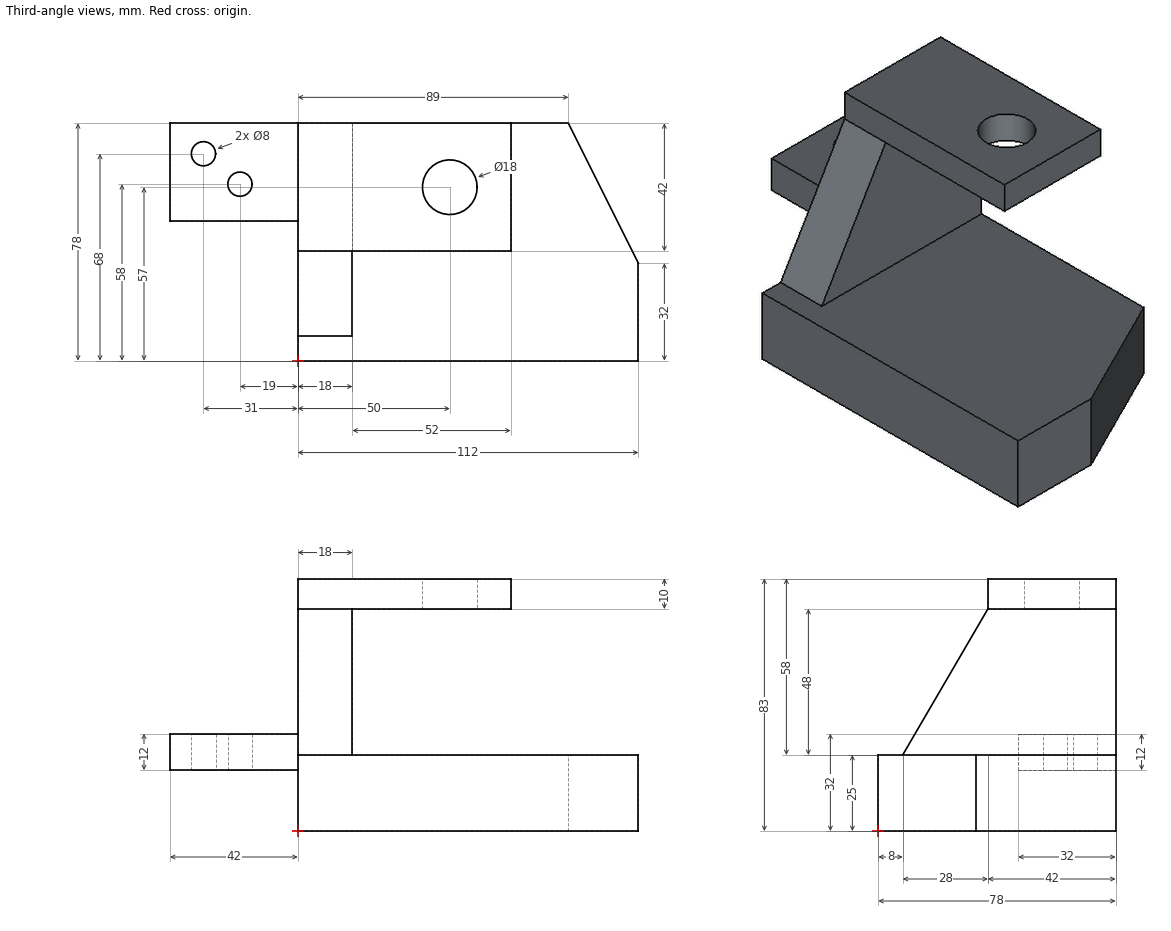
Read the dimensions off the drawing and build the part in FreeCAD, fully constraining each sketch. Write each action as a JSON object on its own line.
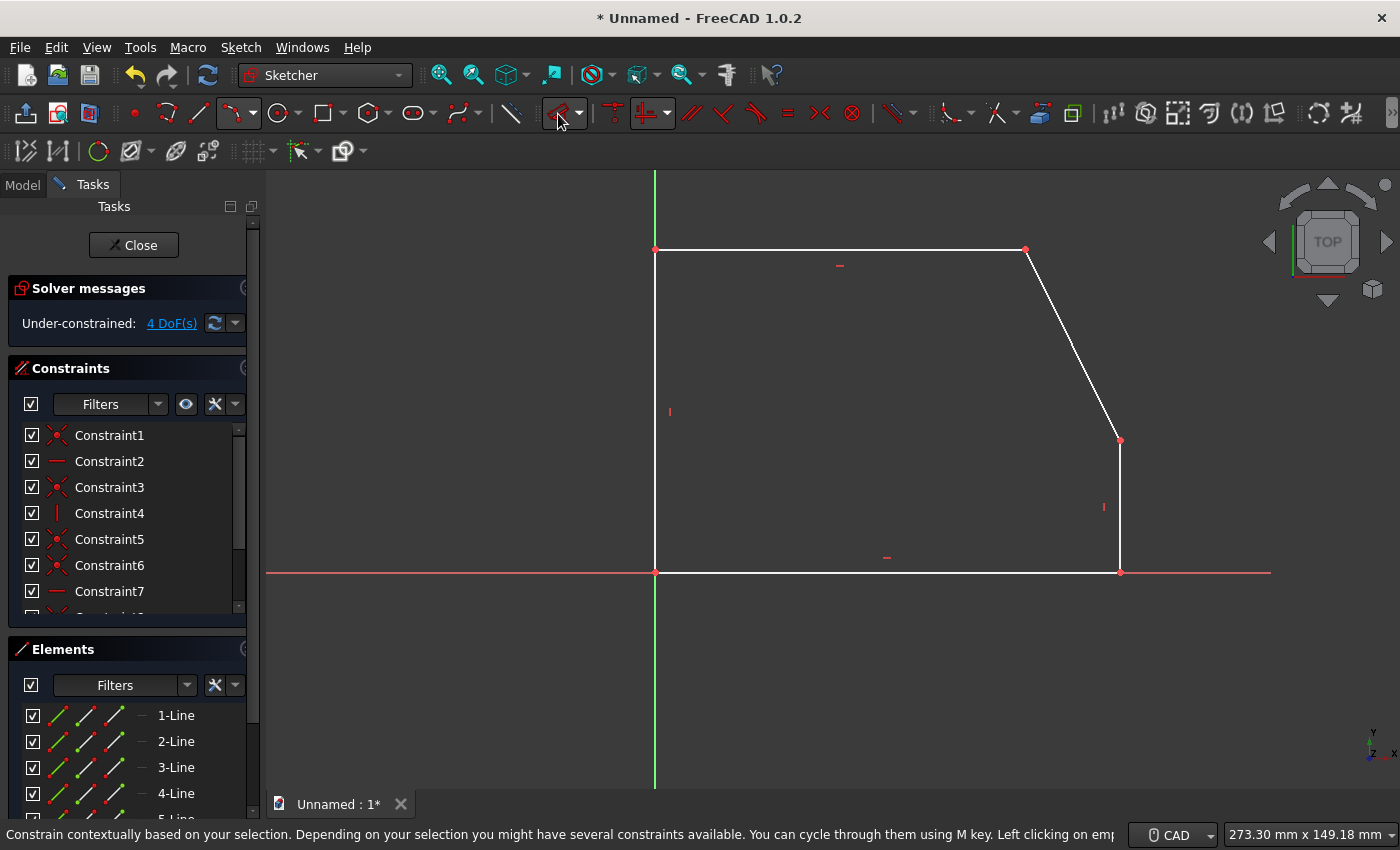
{"action": "left_click", "coordinate": [1120, 533]}
{"action": "left_click", "coordinate": [1154, 507]}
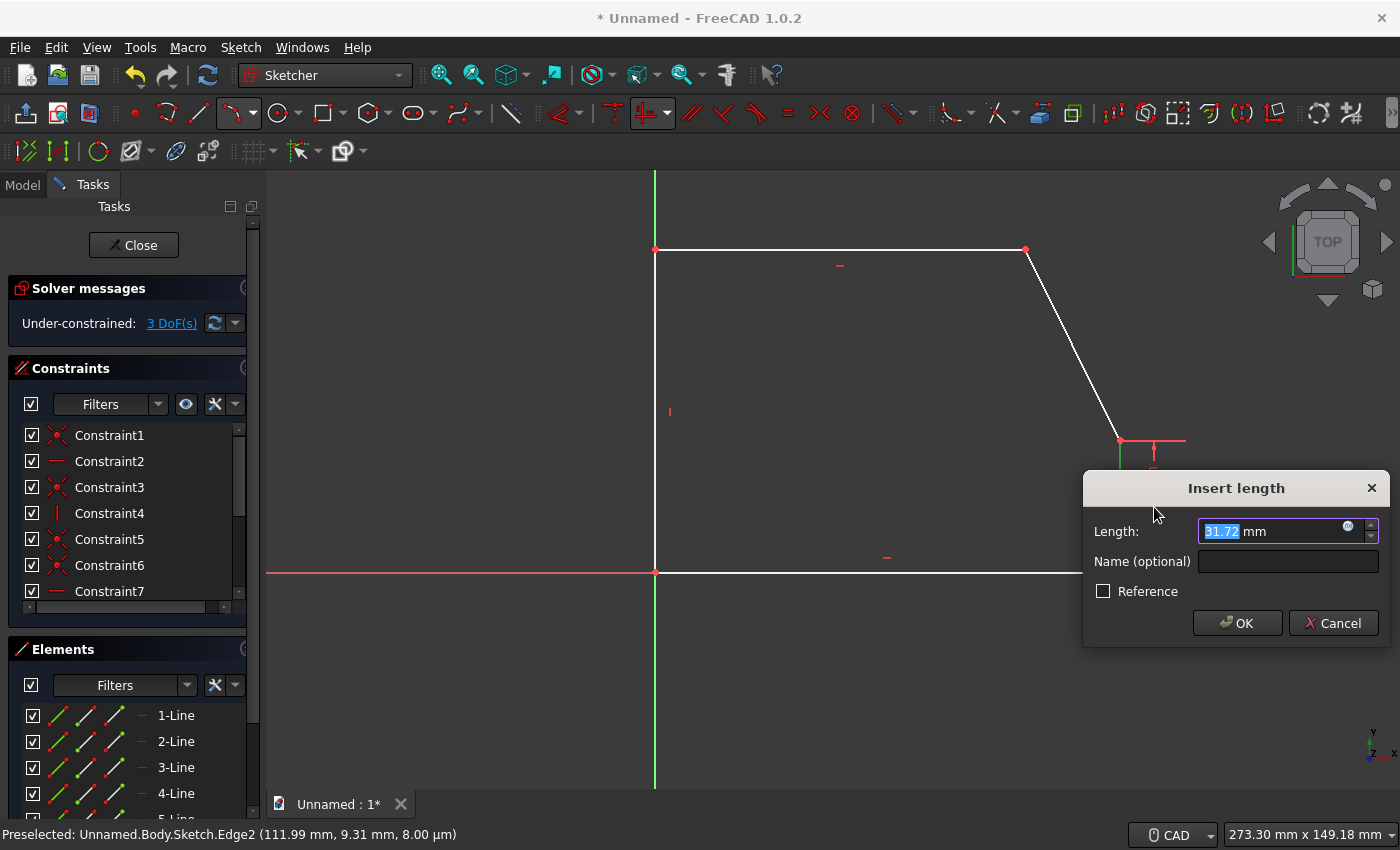
{"action": "type", "text": "32"}
{"action": "key", "text": "Return"}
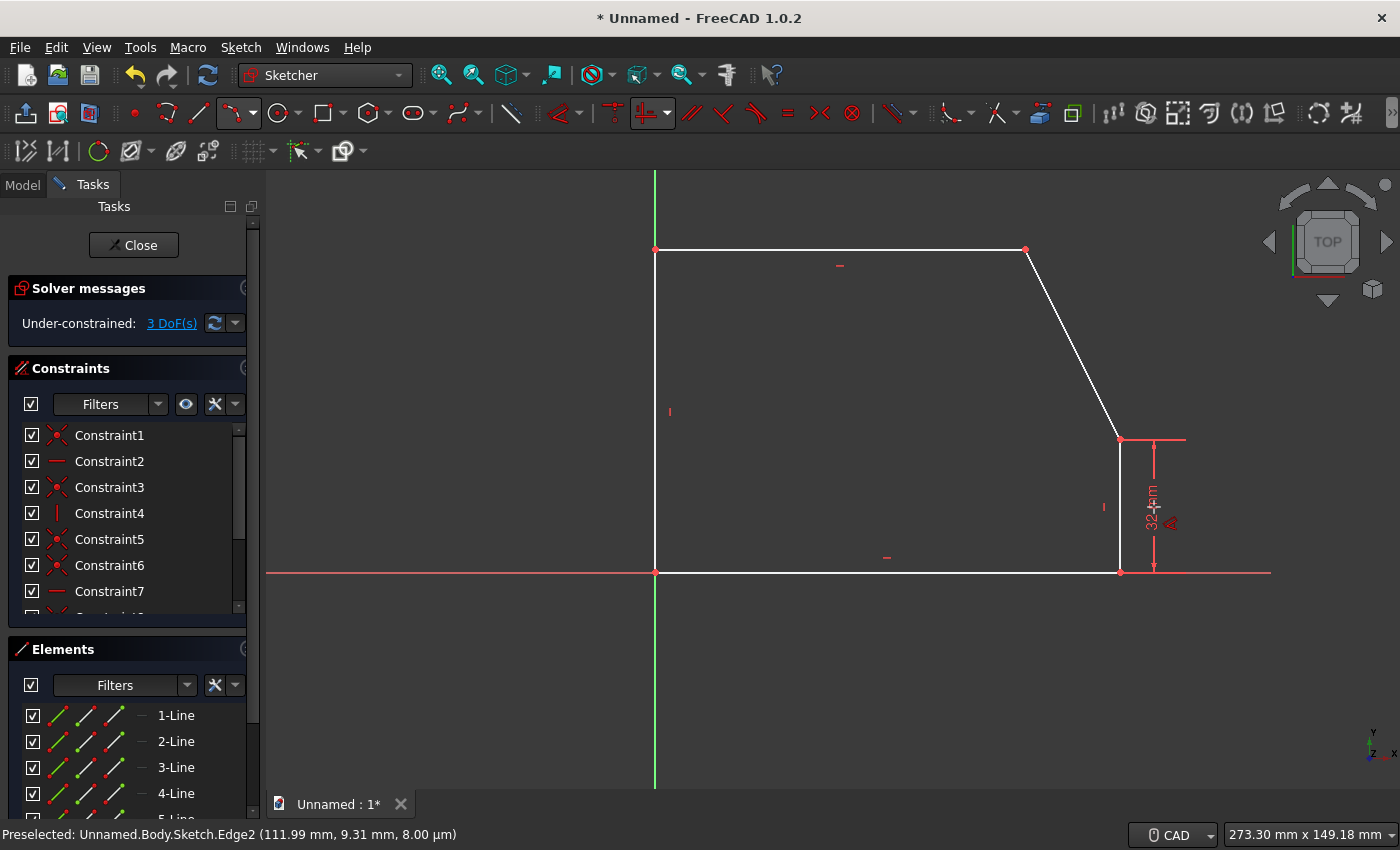
{"action": "left_click", "coordinate": [914, 250]}
{"action": "left_click", "coordinate": [840, 216]}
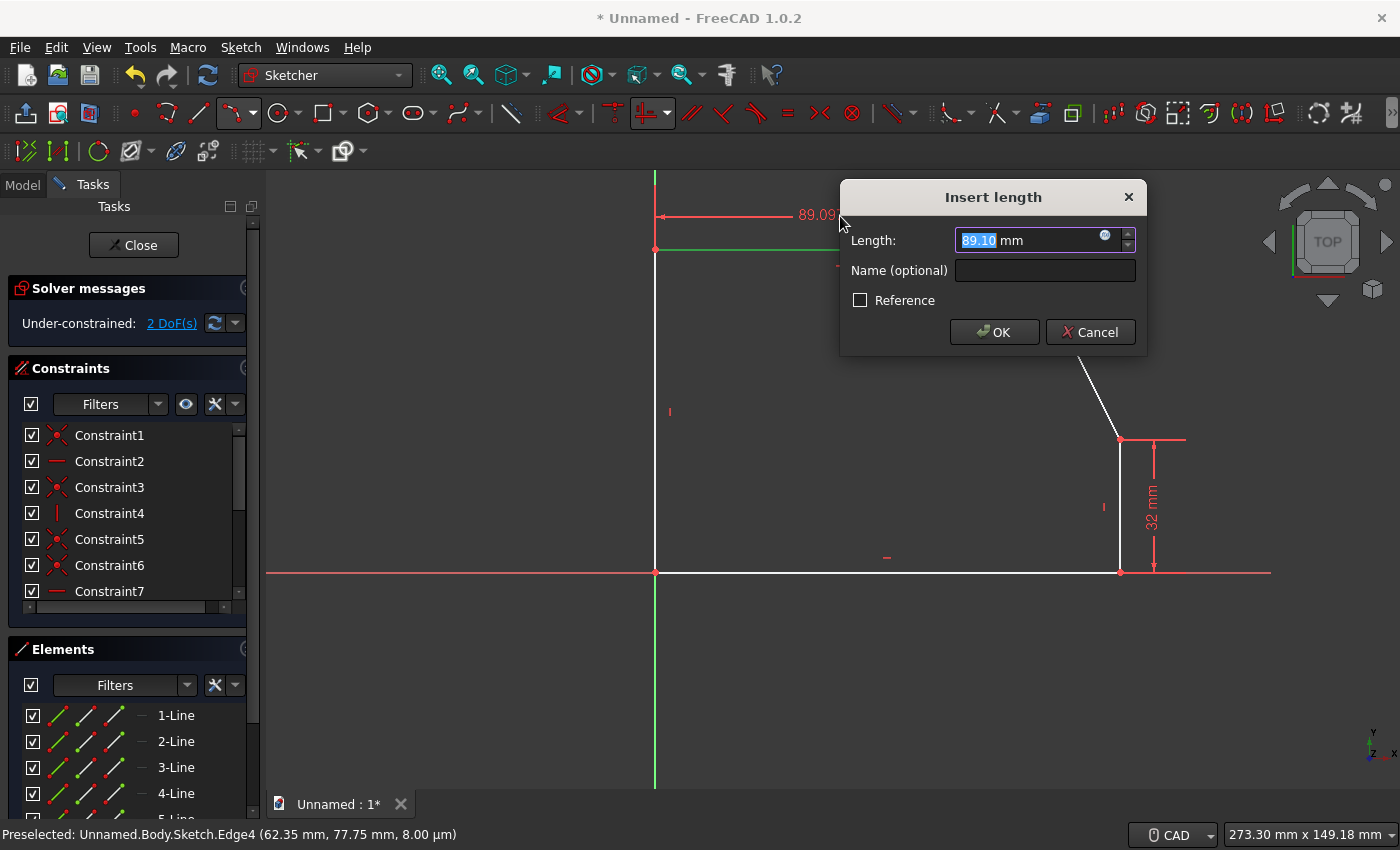
{"action": "type", "text": "89"}
{"action": "key", "text": "Return"}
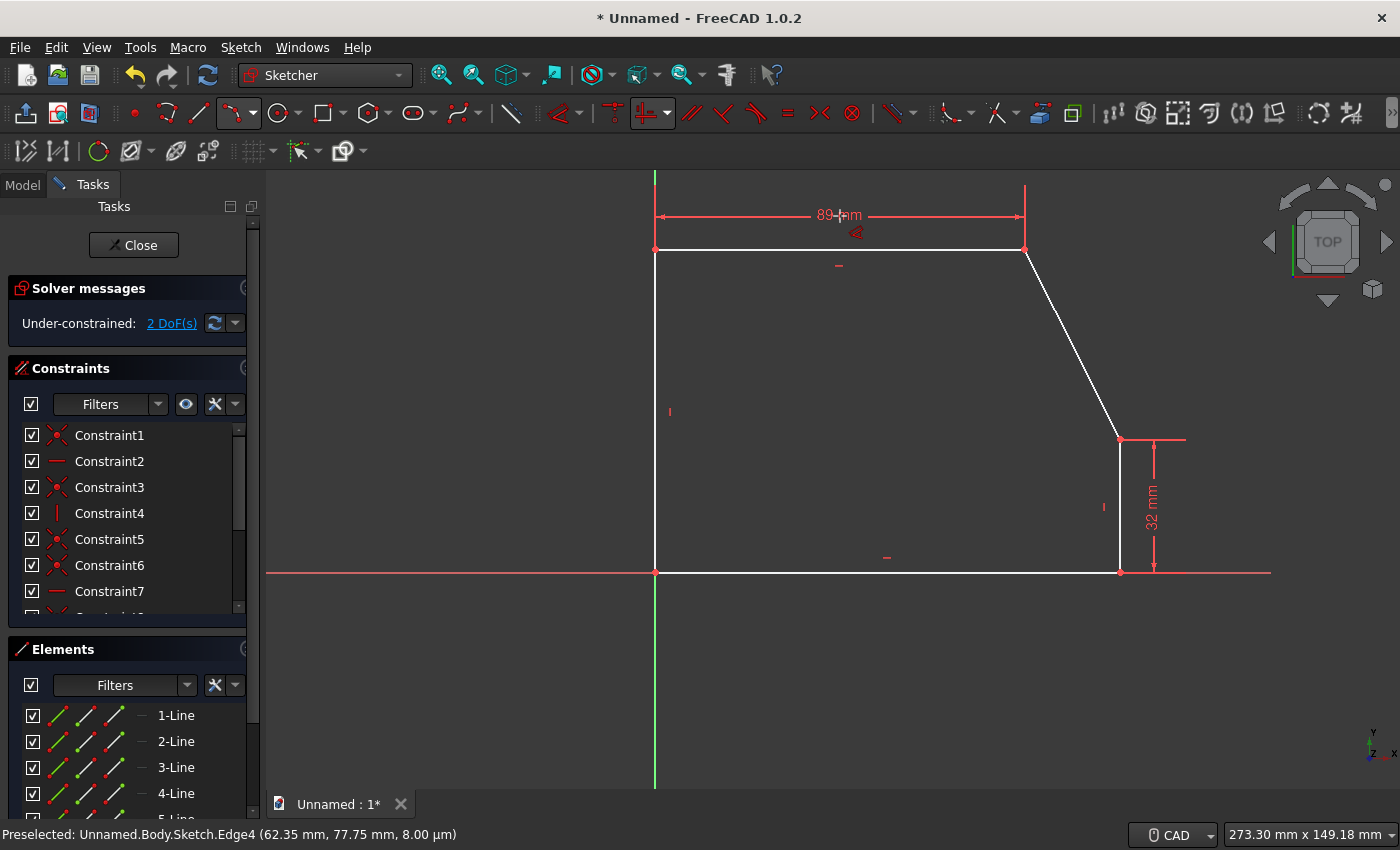
{"action": "left_click", "coordinate": [655, 347]}
{"action": "left_click", "coordinate": [621, 411]}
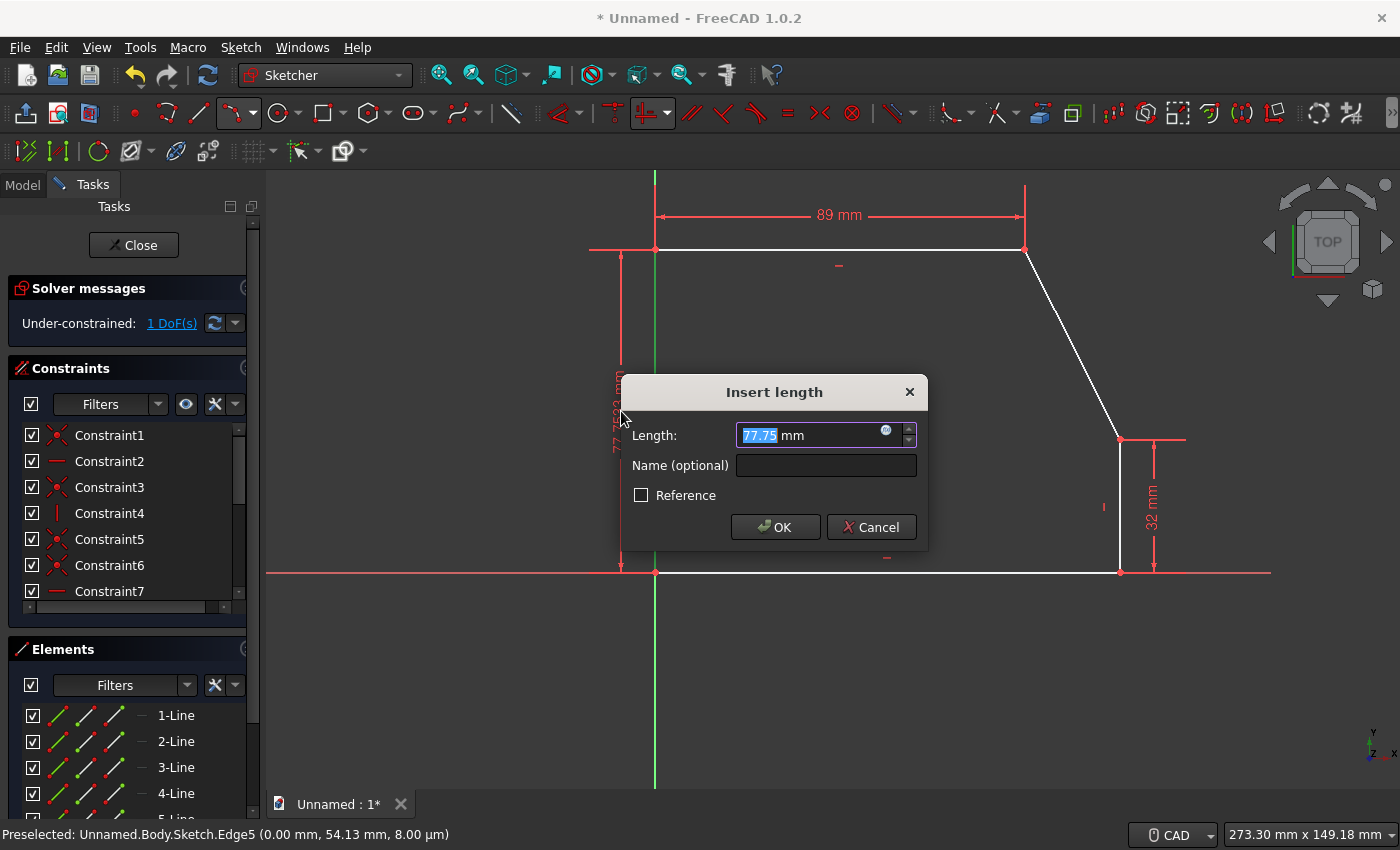
{"action": "type", "text": "78"}
{"action": "key", "text": "Return"}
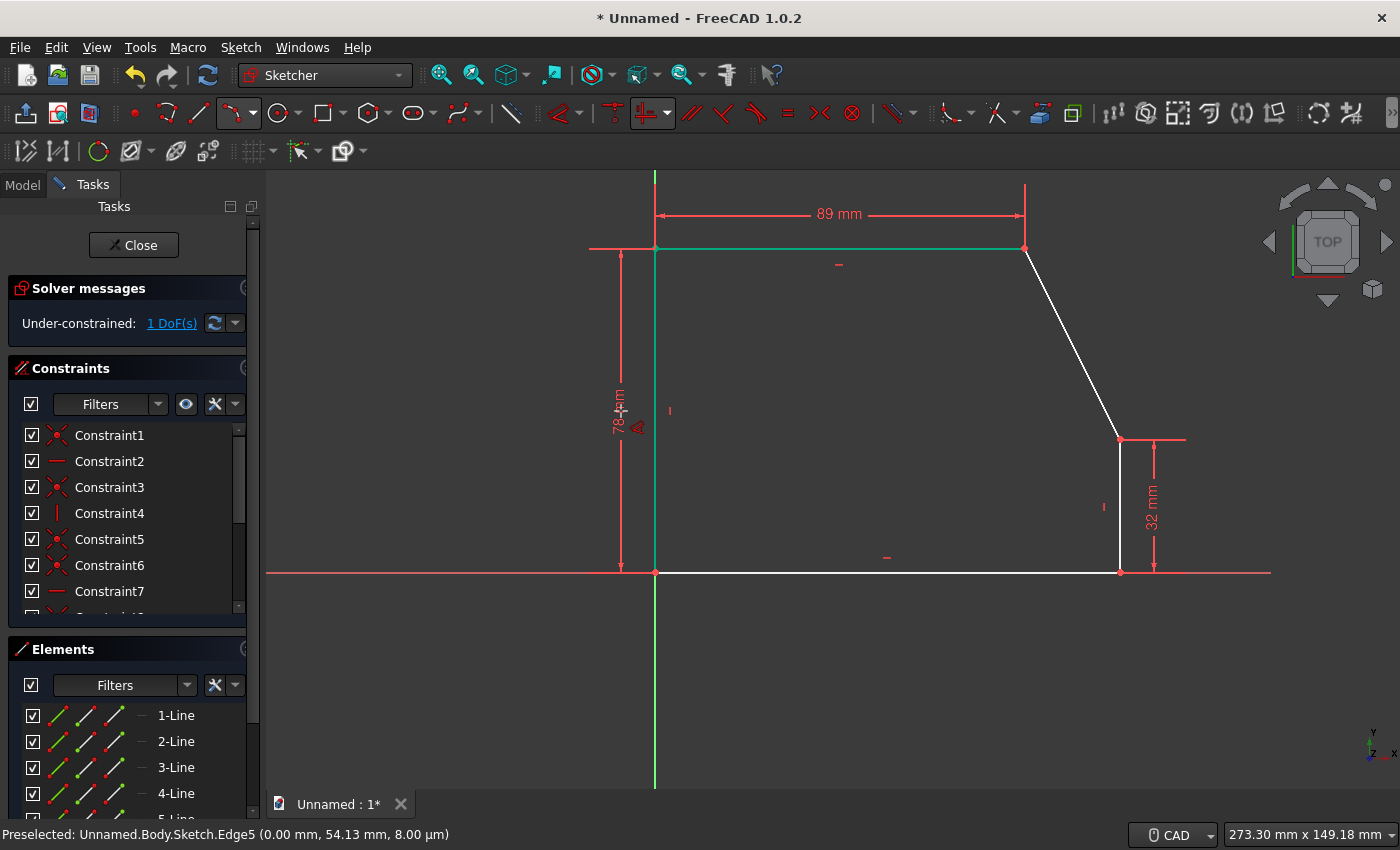
{"action": "left_click", "coordinate": [795, 573]}
{"action": "left_click", "coordinate": [888, 607]}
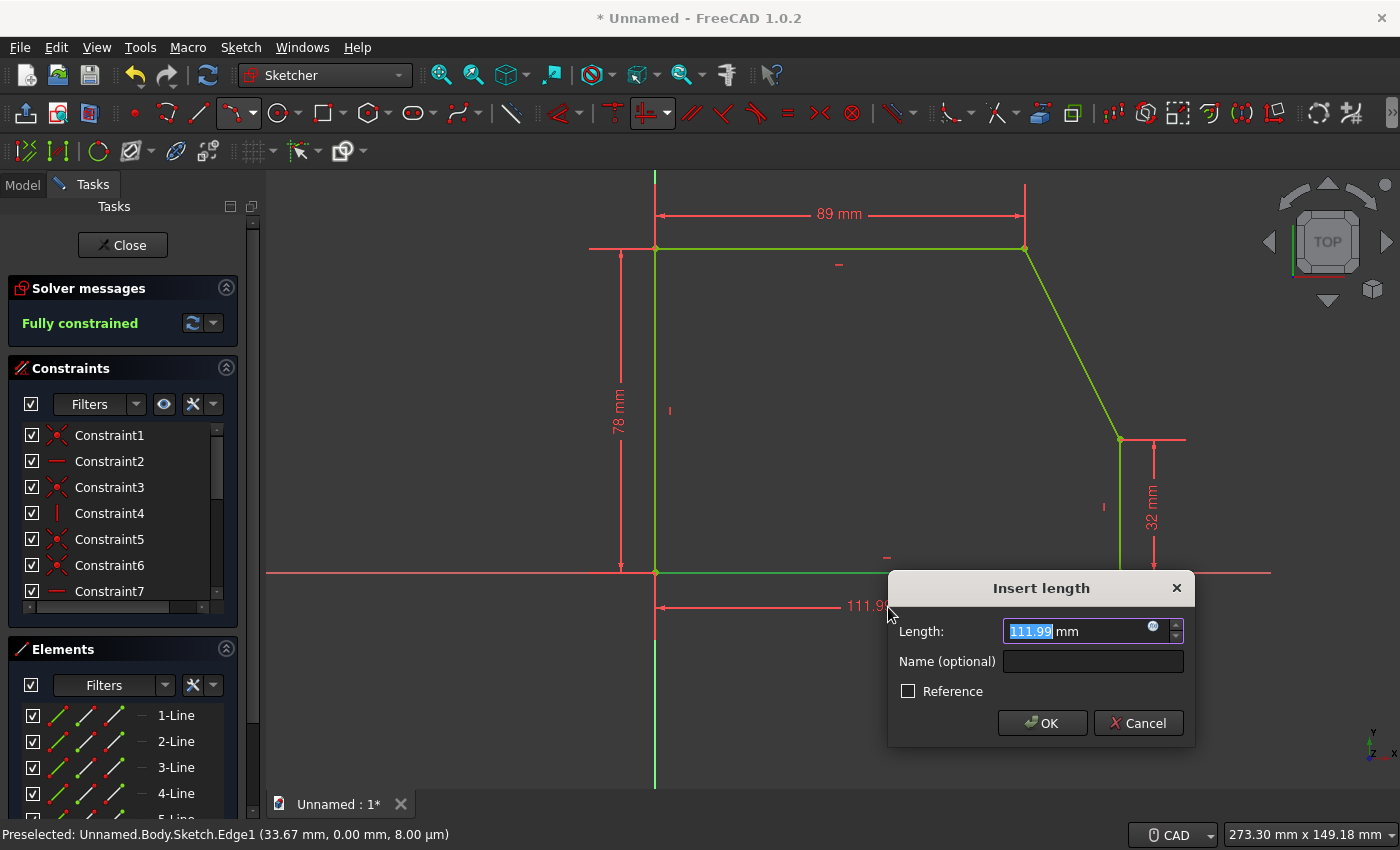
{"action": "type", "text": "112"}
{"action": "key", "text": "Return"}
{"action": "key", "text": "Escape"}